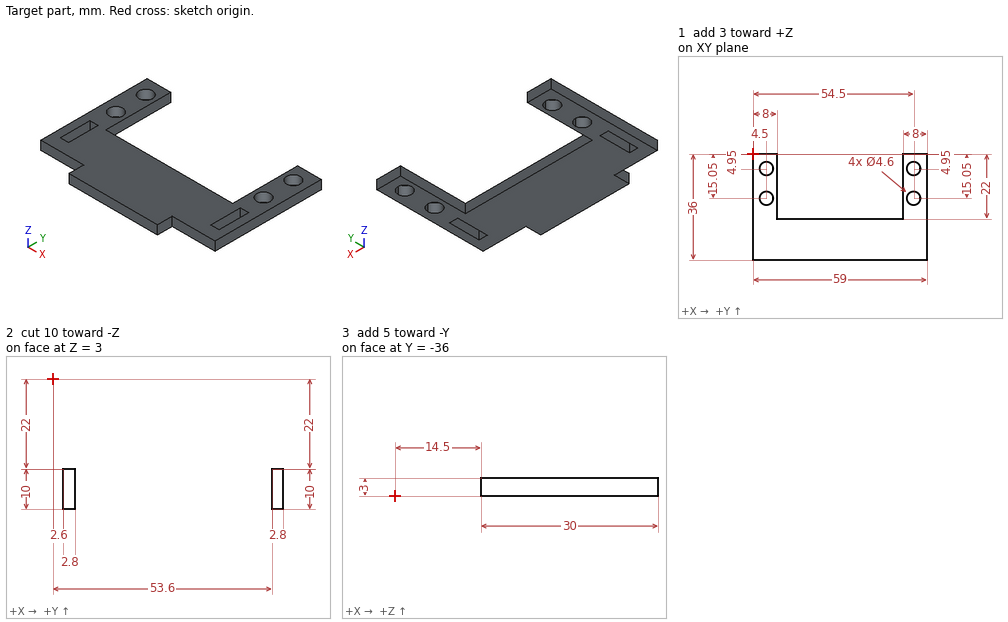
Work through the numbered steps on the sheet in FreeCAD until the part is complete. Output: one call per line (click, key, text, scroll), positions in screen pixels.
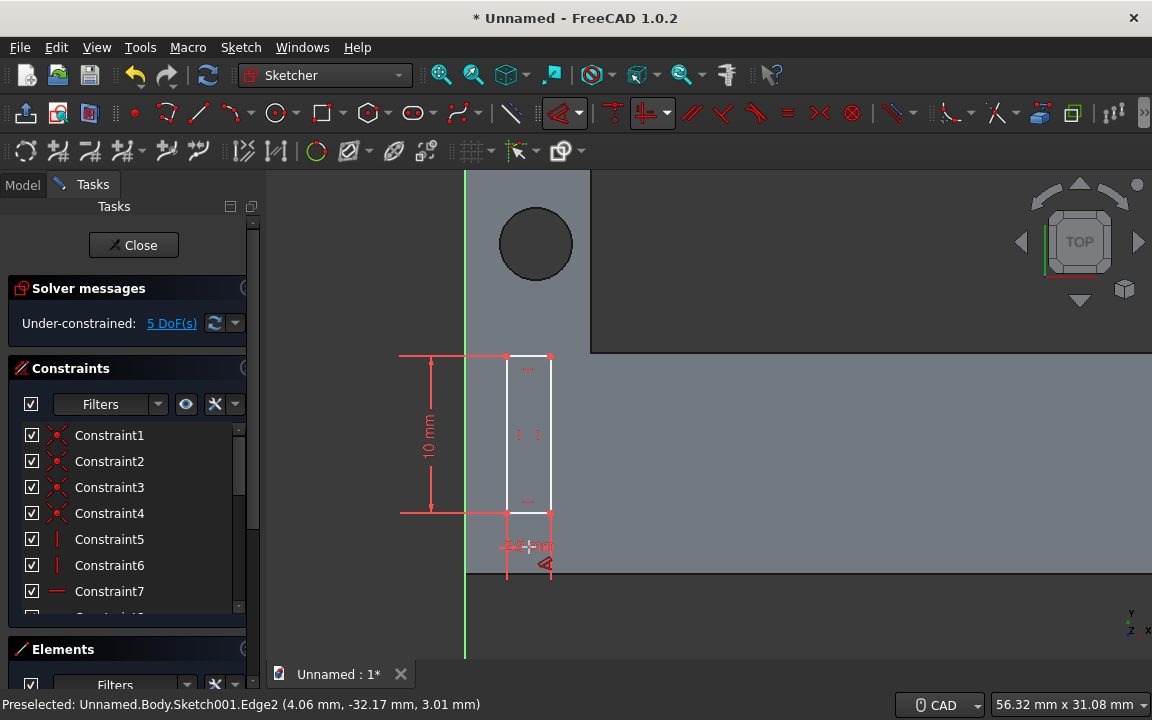
scroll(314, 604, down, 3)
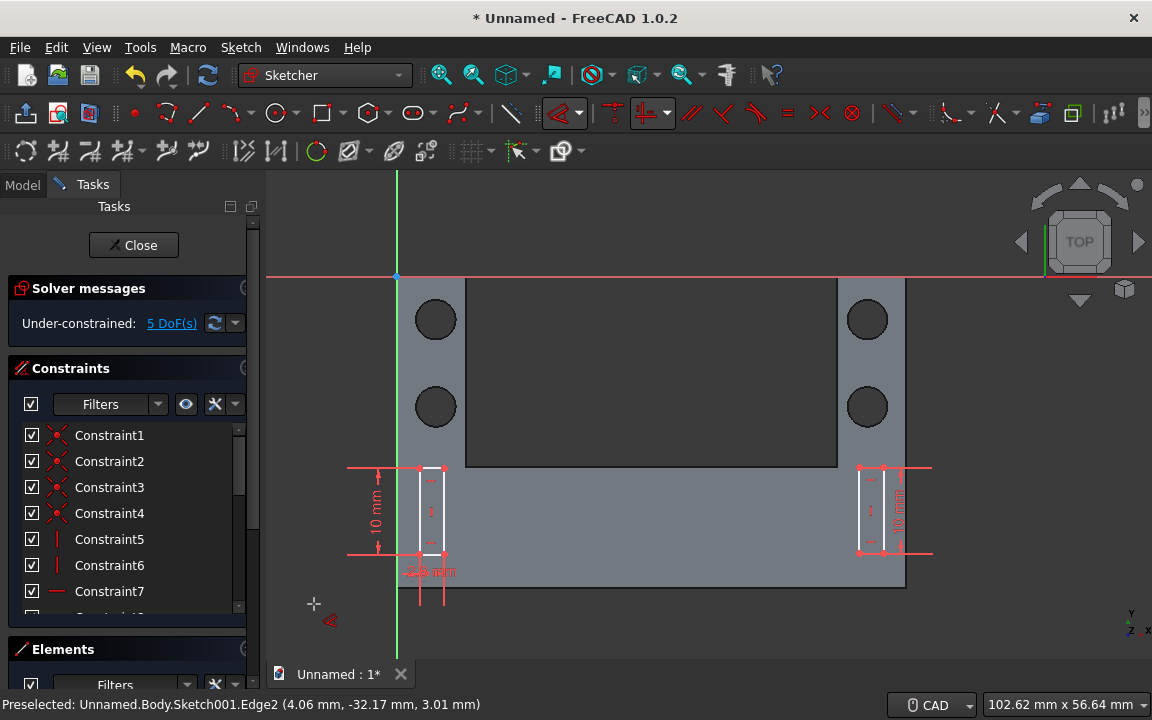
scroll(867, 554, up, 4)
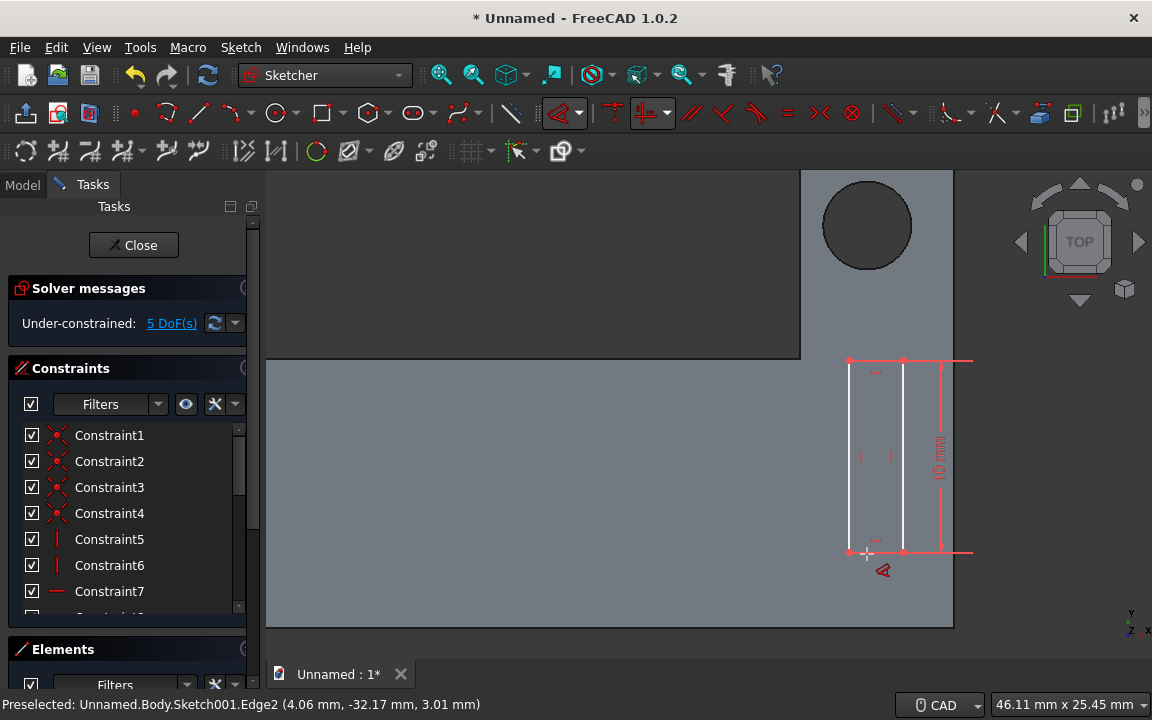
click(865, 553)
click(876, 587)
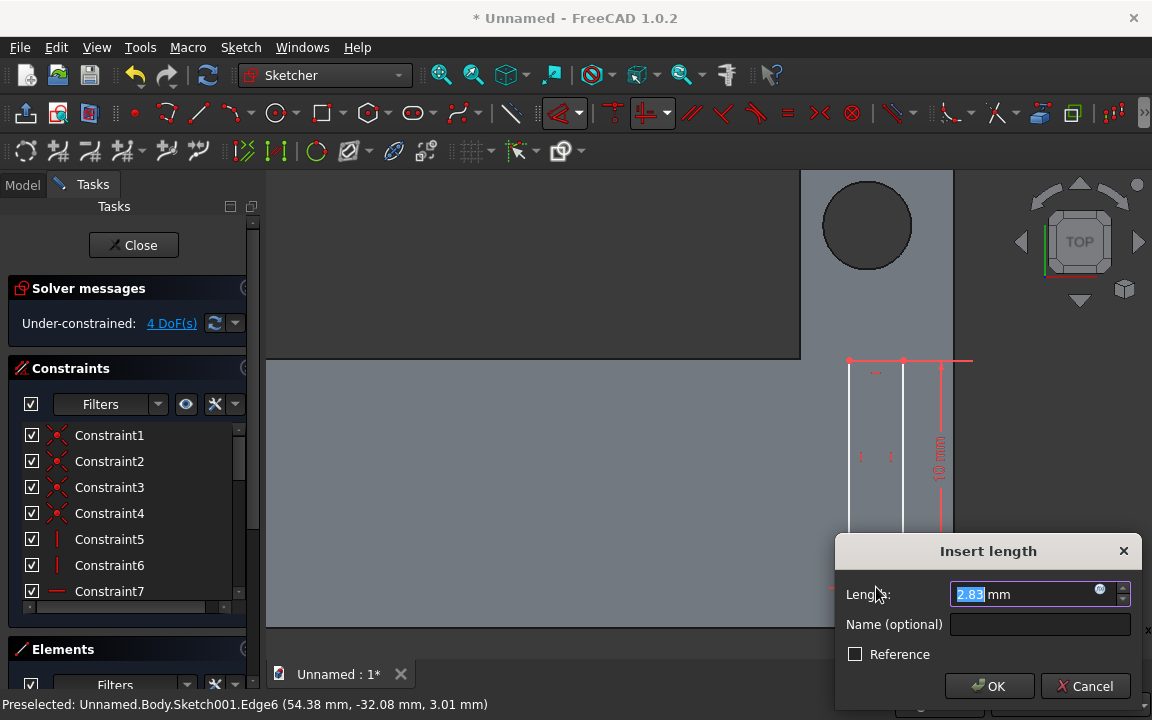
text(2.8)
key(Return)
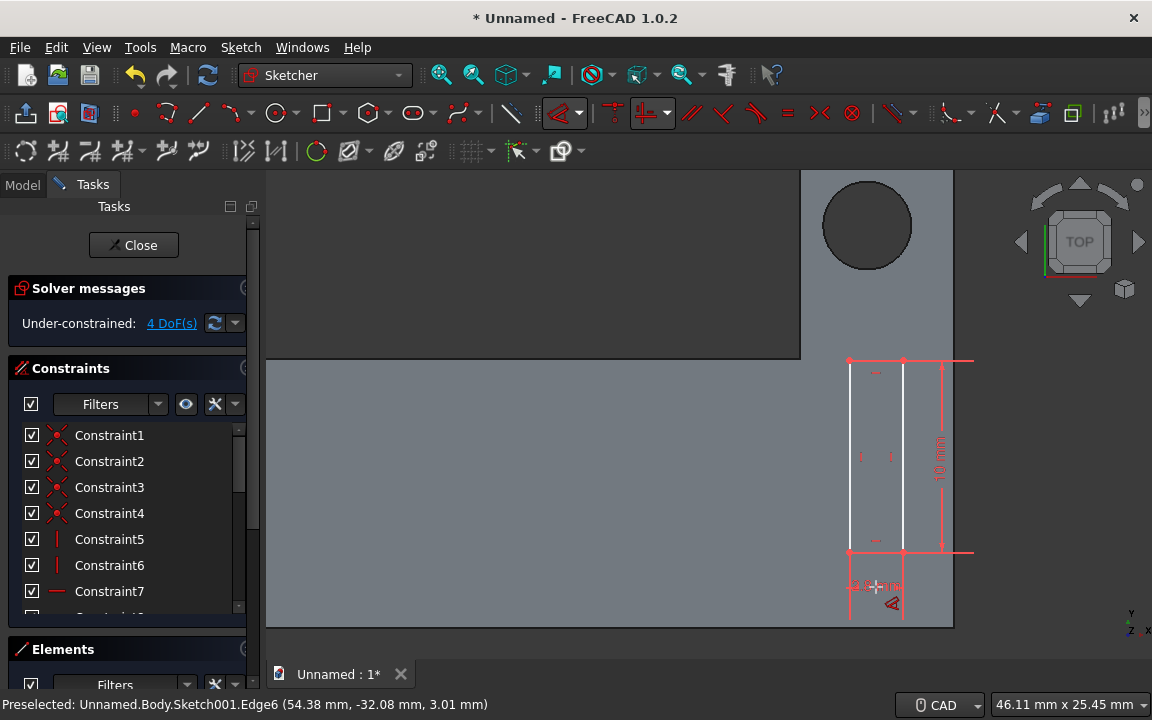
scroll(868, 554, down, 4)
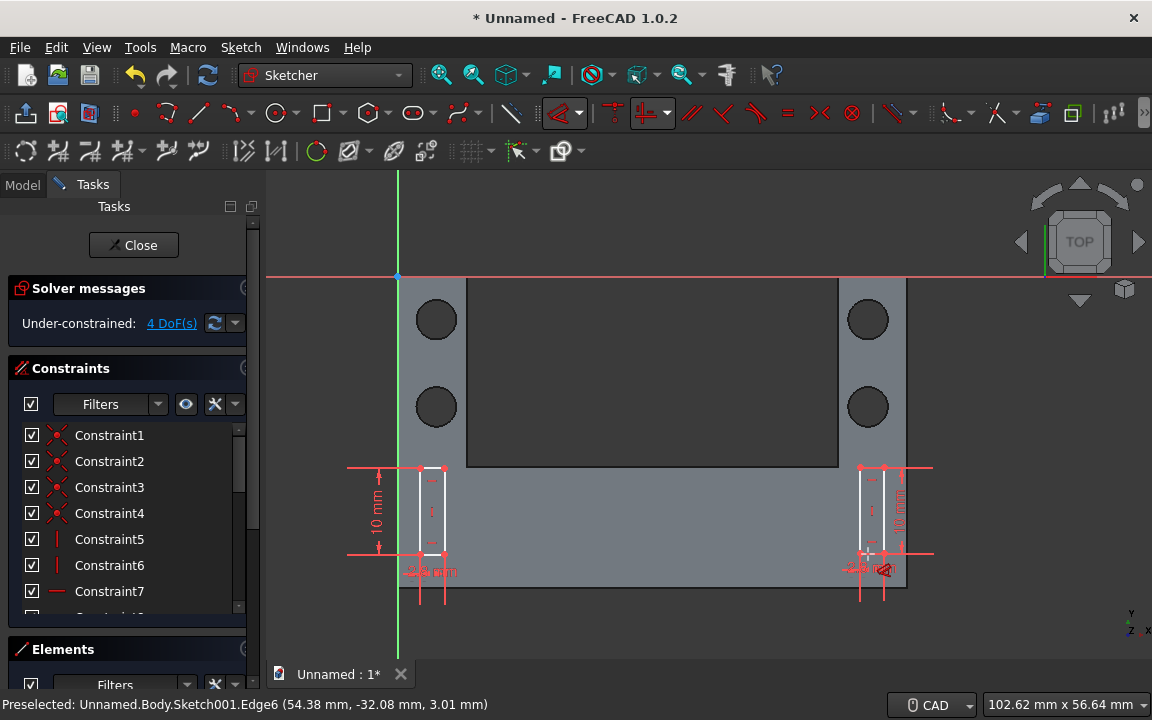
click(420, 468)
click(364, 373)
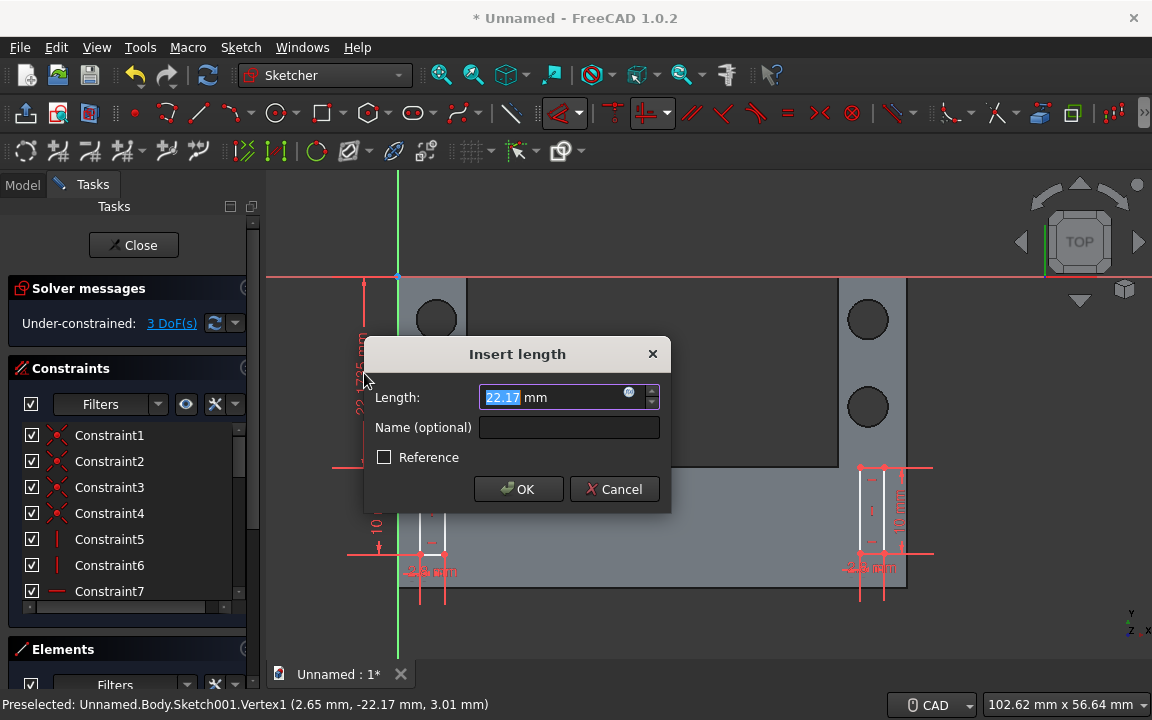
text(22)
key(Return)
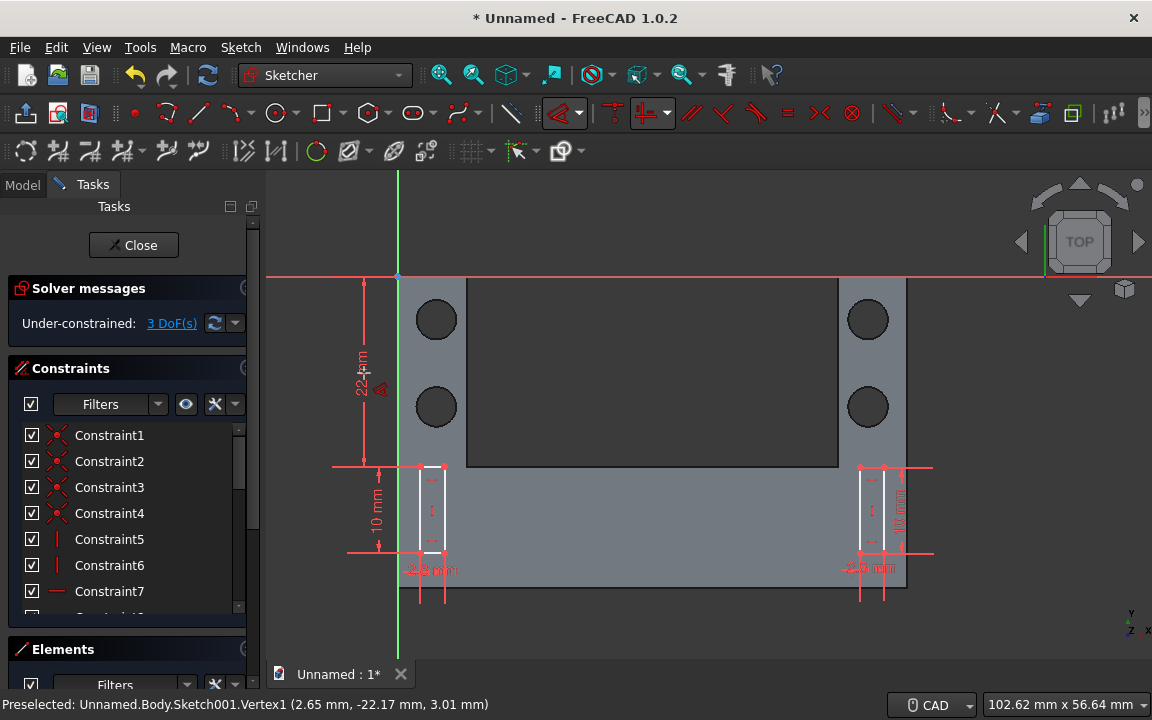
click(860, 468)
click(364, 328)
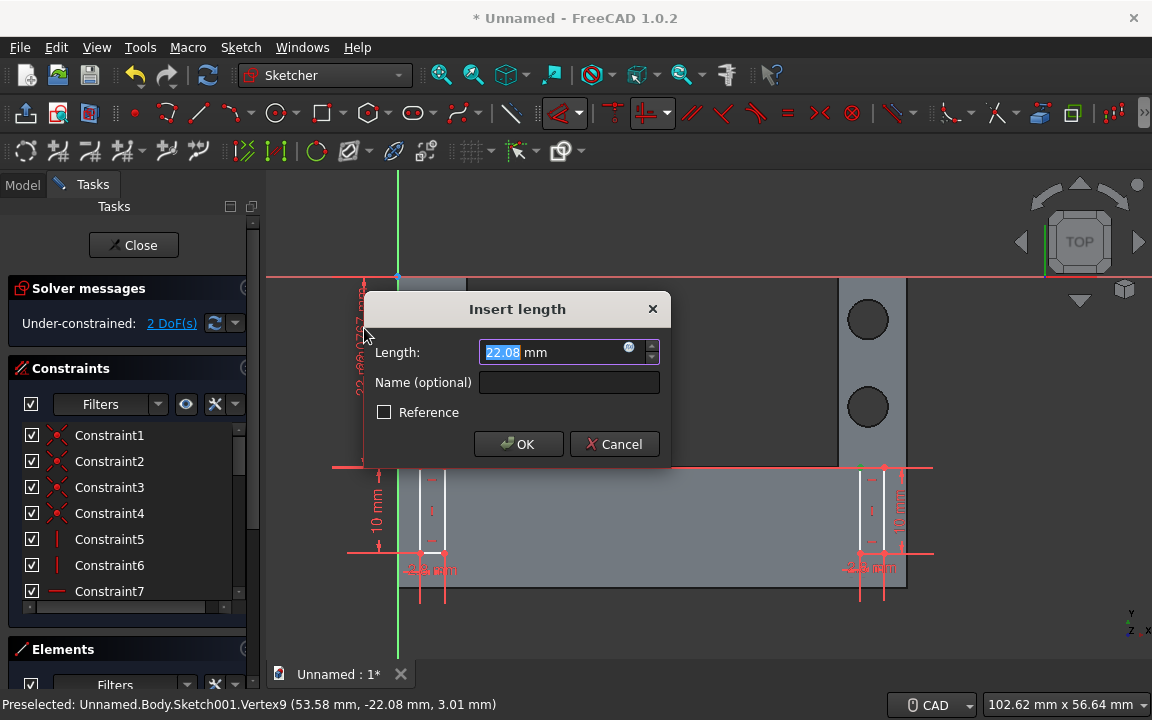
text(22)
key(Return)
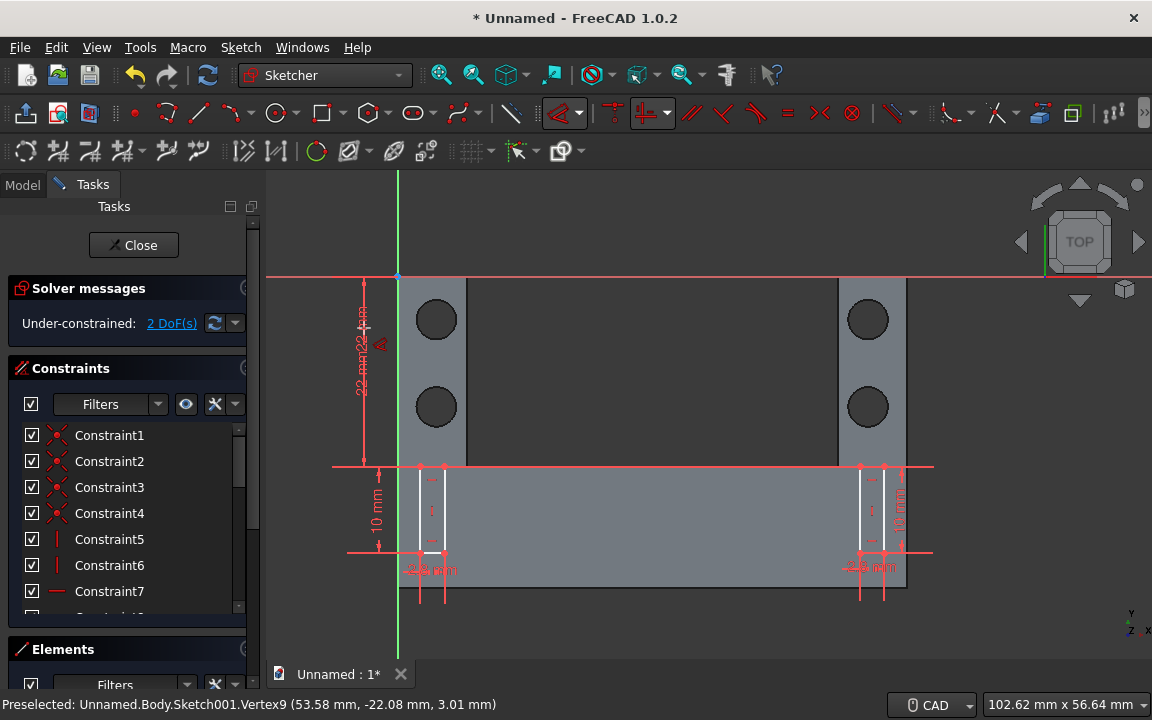
scroll(420, 467, up, 3)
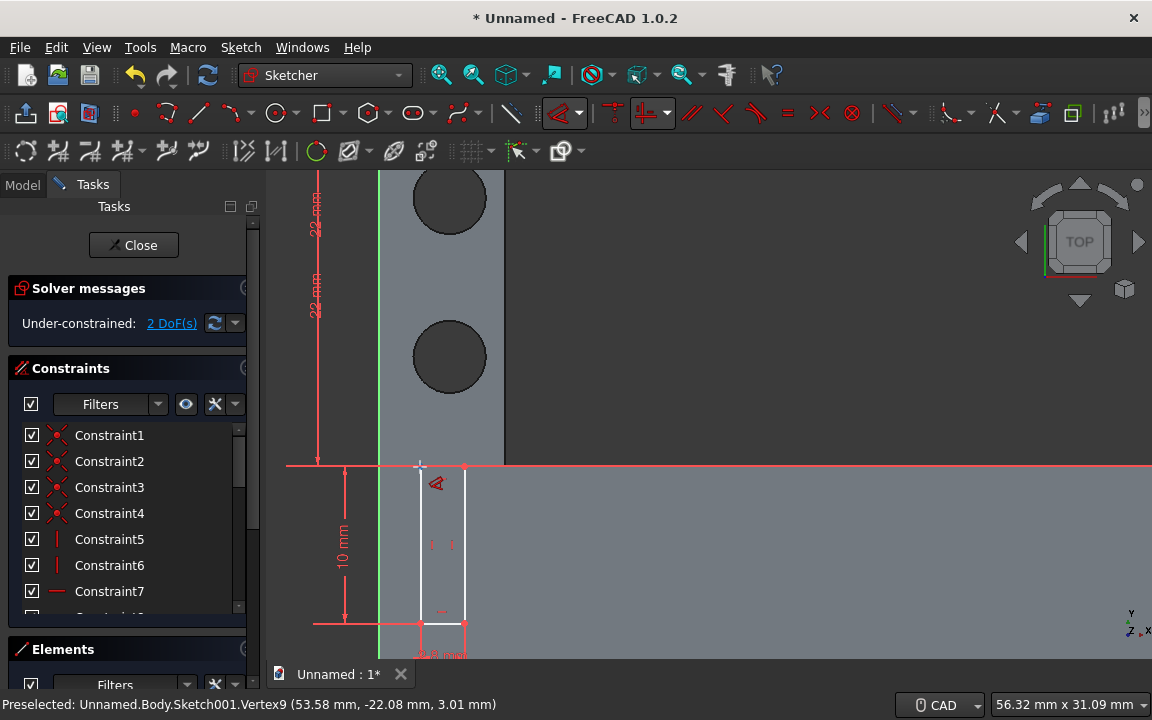
click(421, 466)
click(400, 500)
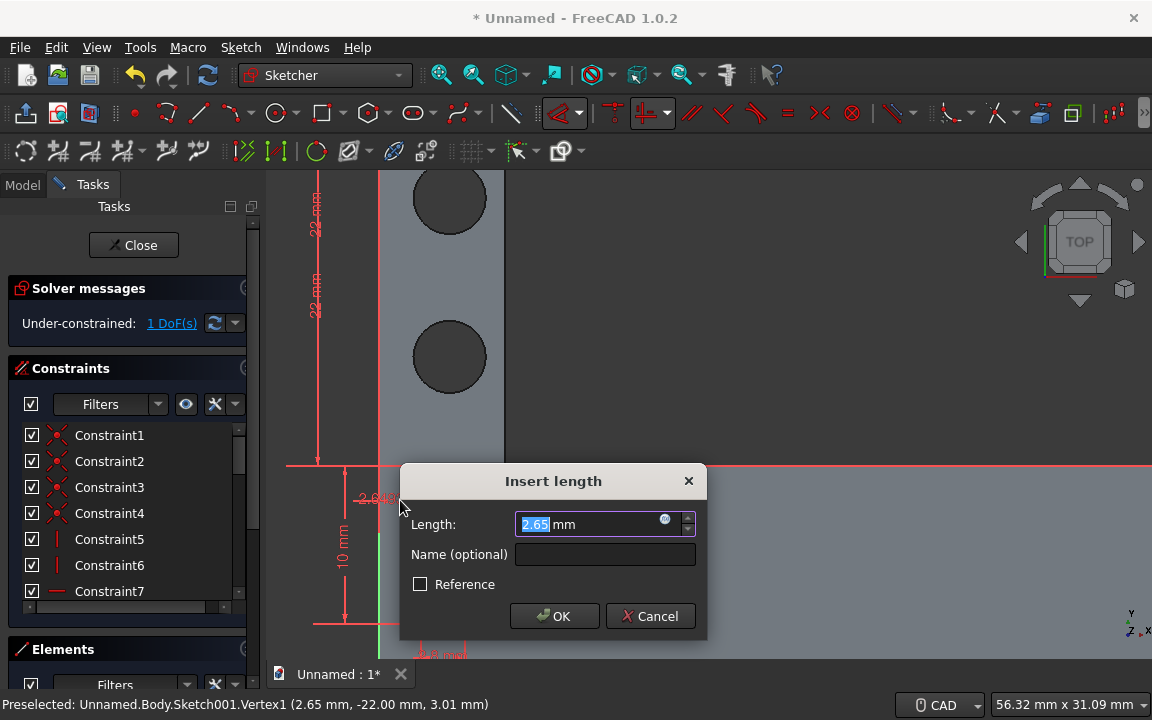
text(2.6)
key(Return)